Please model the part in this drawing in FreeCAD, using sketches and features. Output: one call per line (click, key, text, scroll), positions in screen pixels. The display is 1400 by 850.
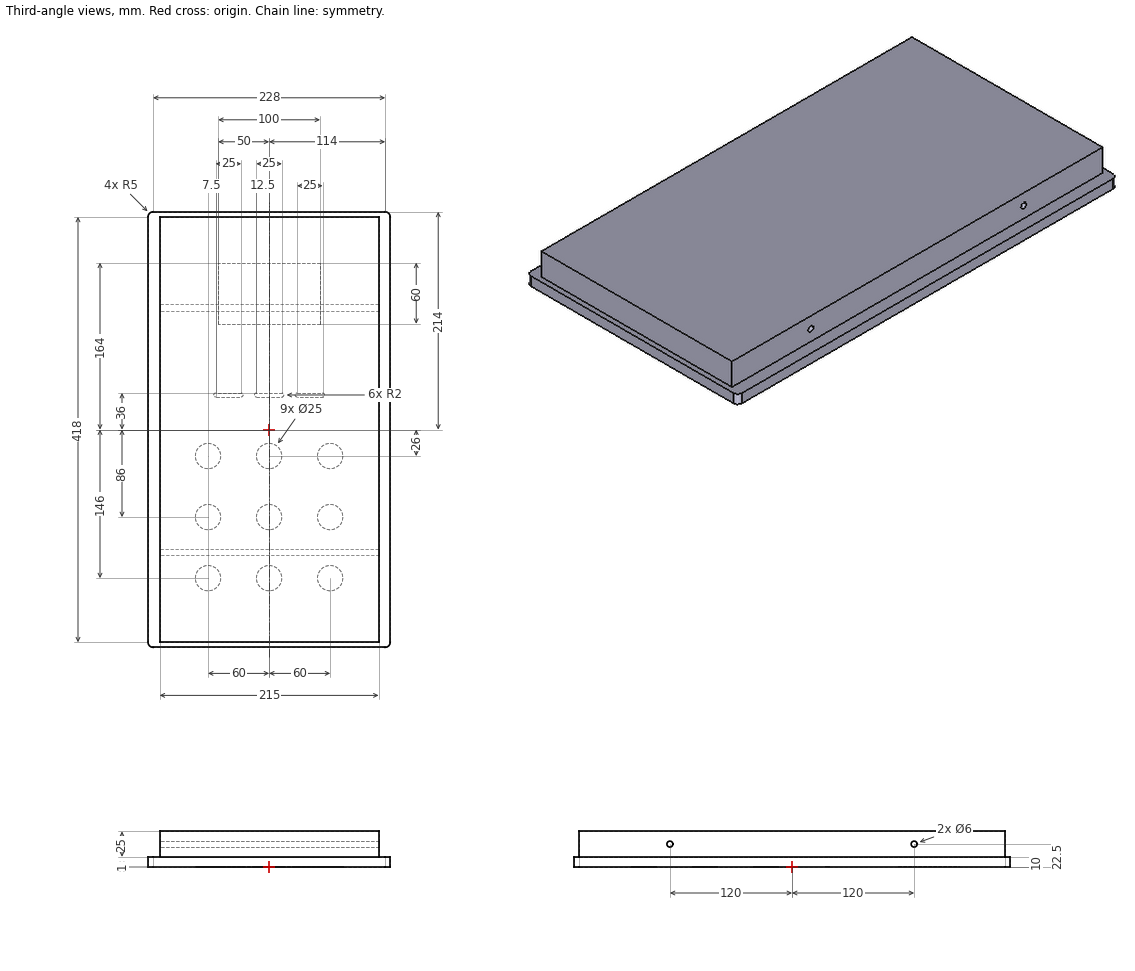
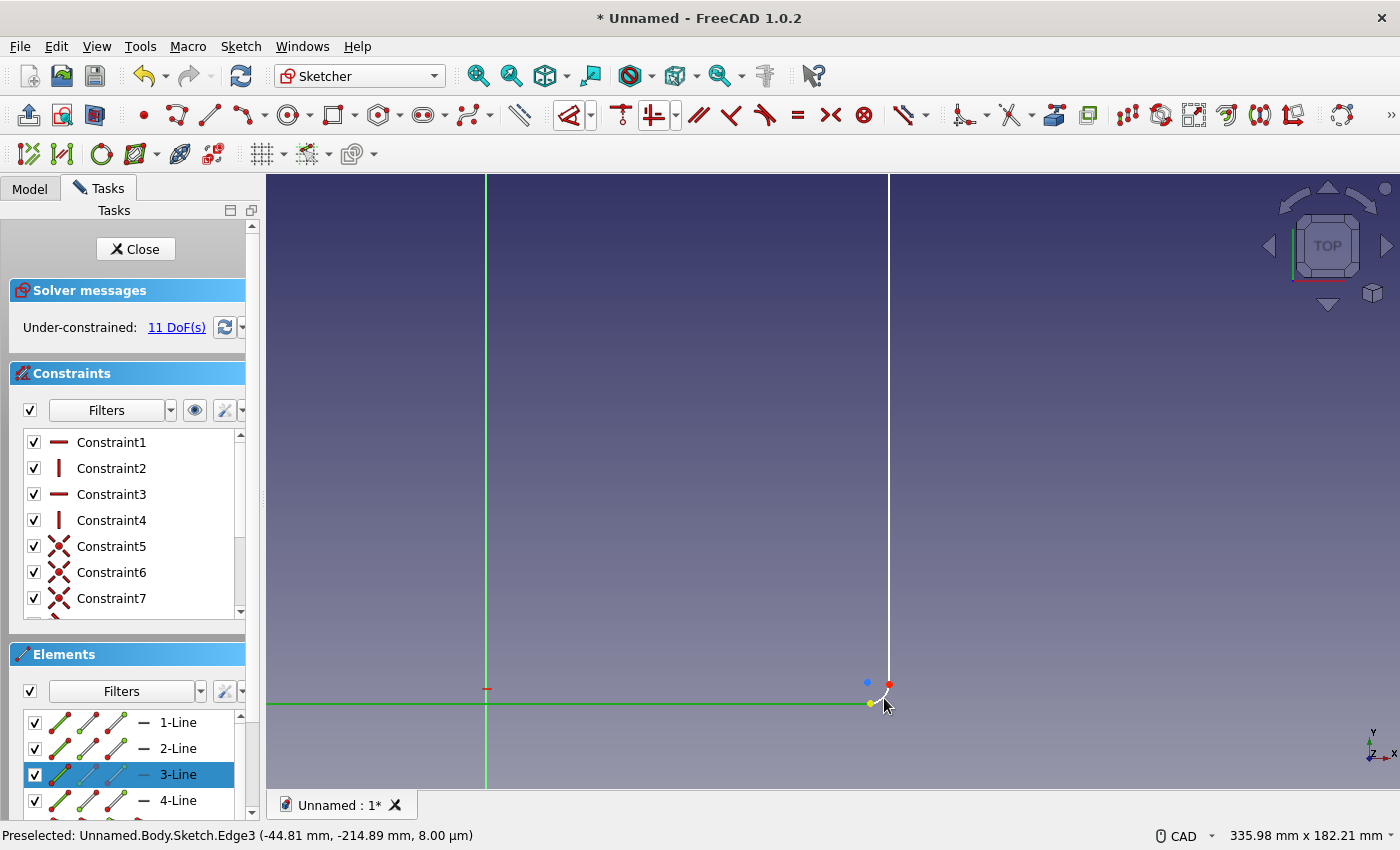
click(883, 698)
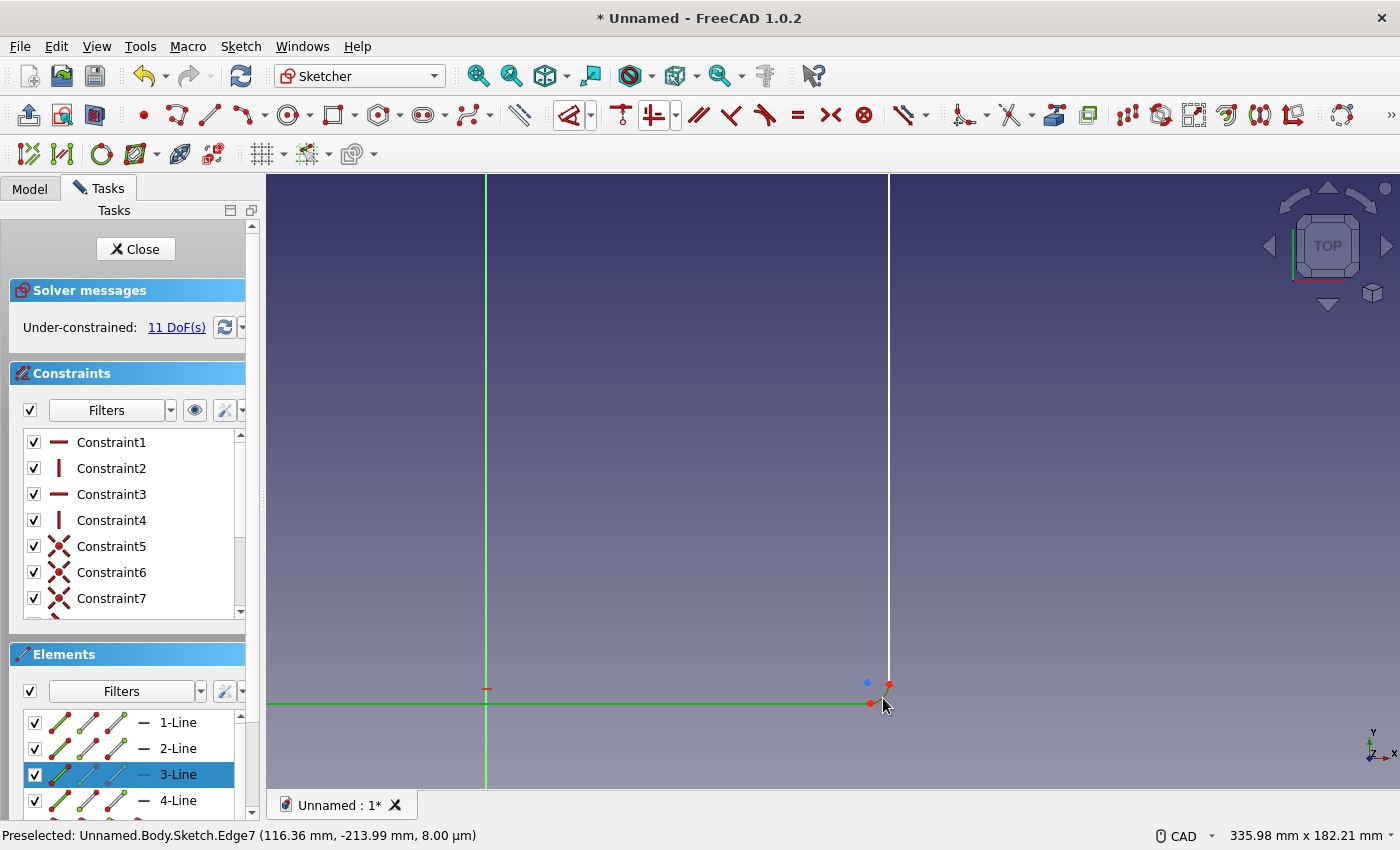
click(765, 116)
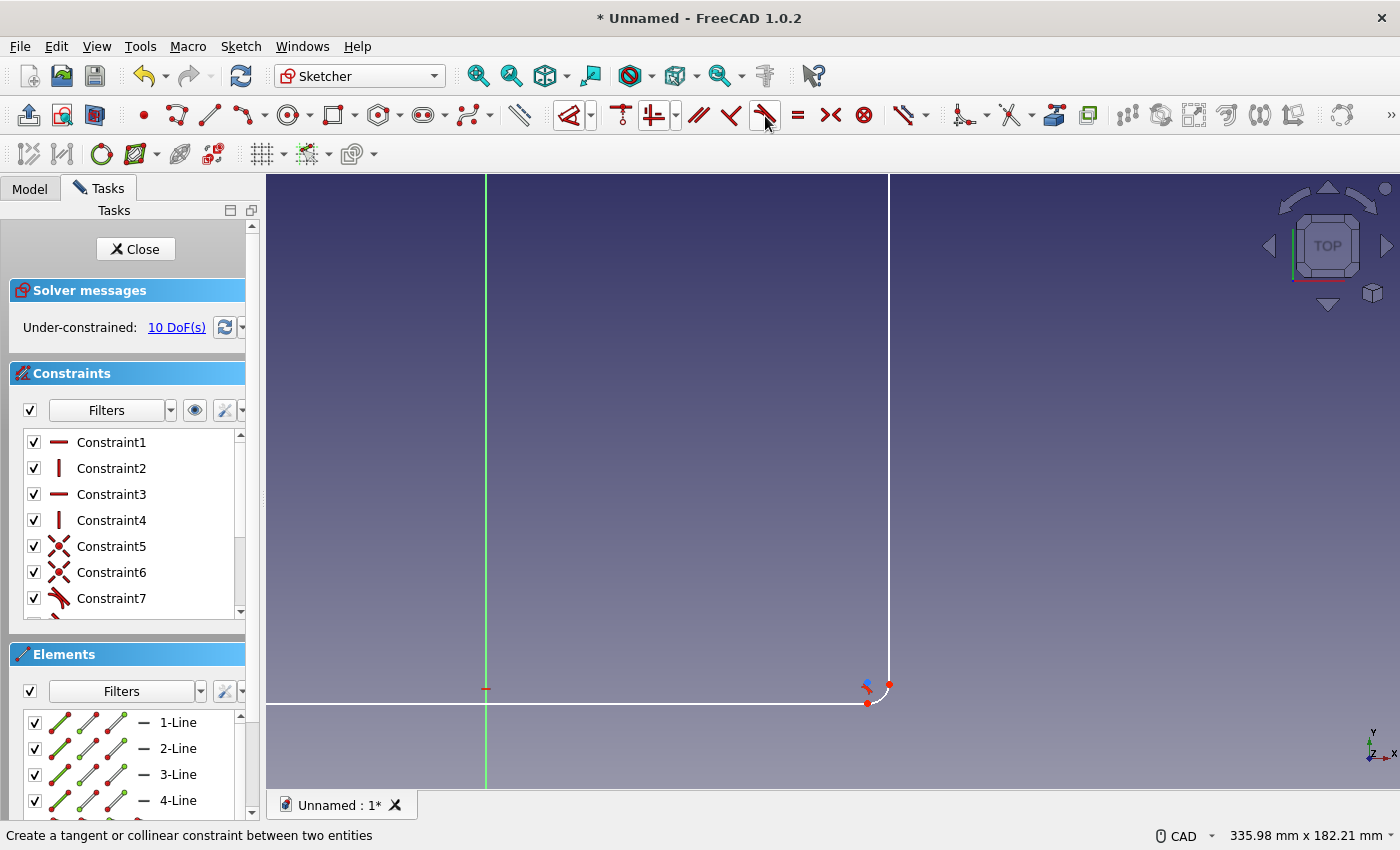
click(889, 262)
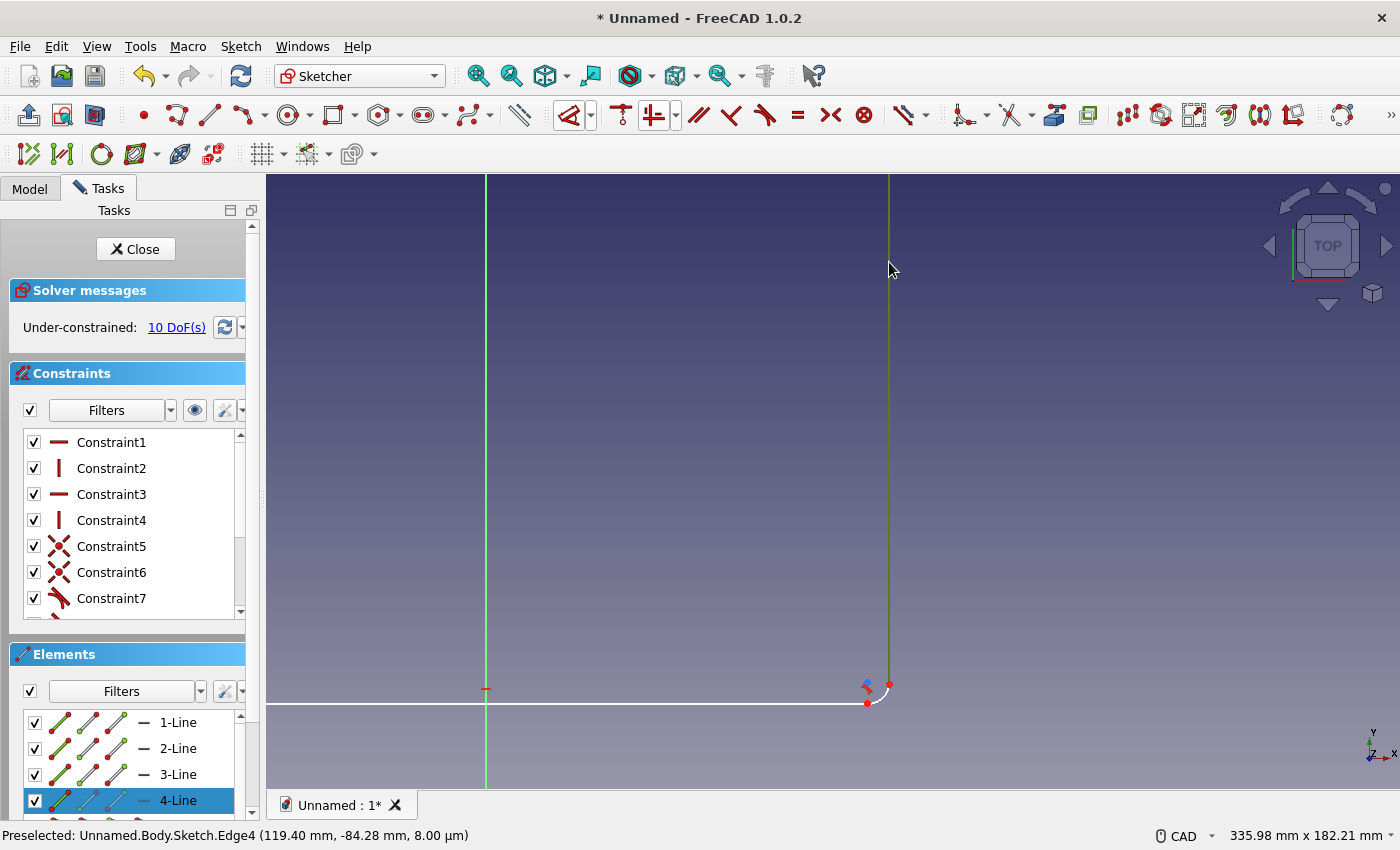
scroll(877, 702, up, 2)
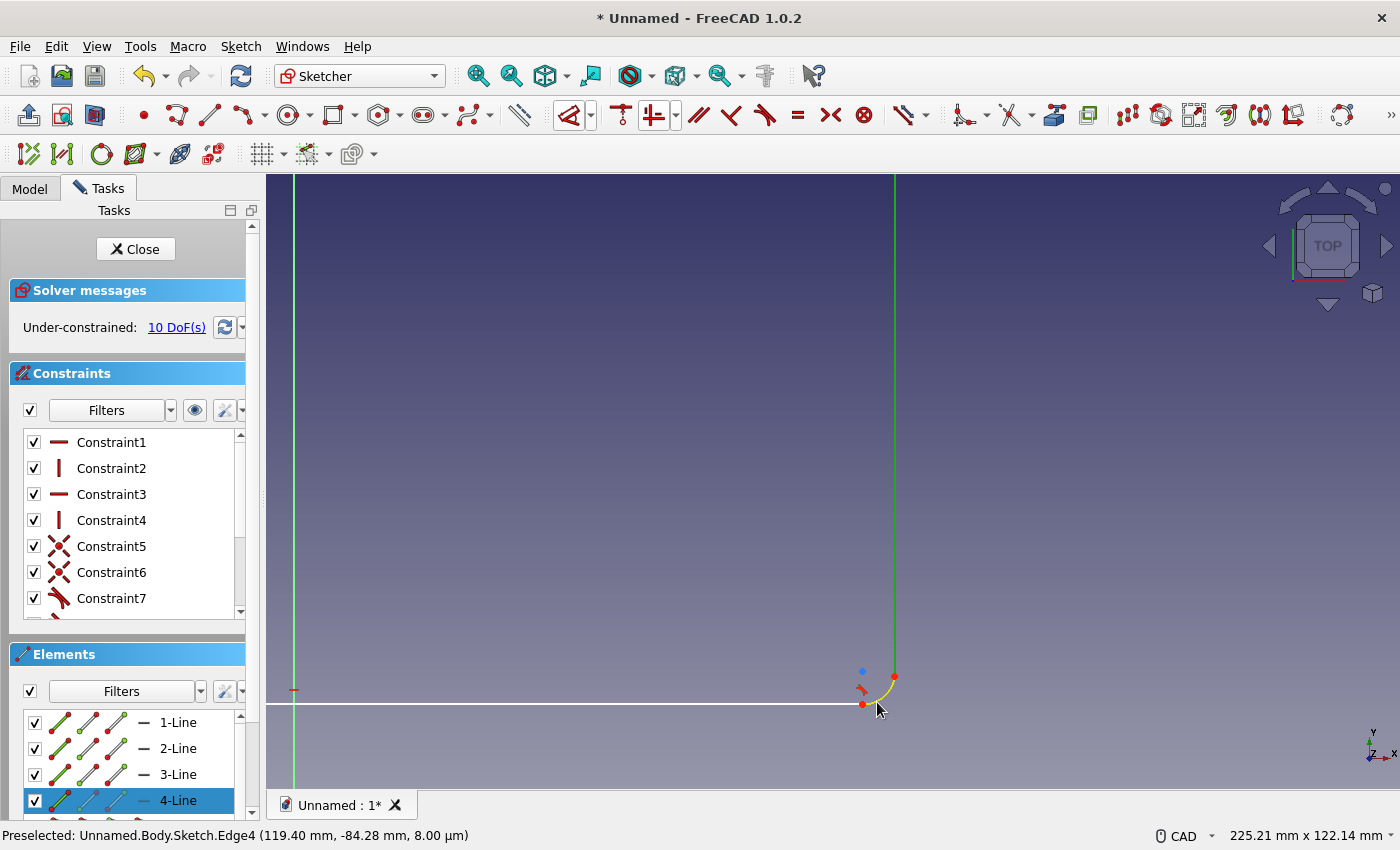
click(876, 701)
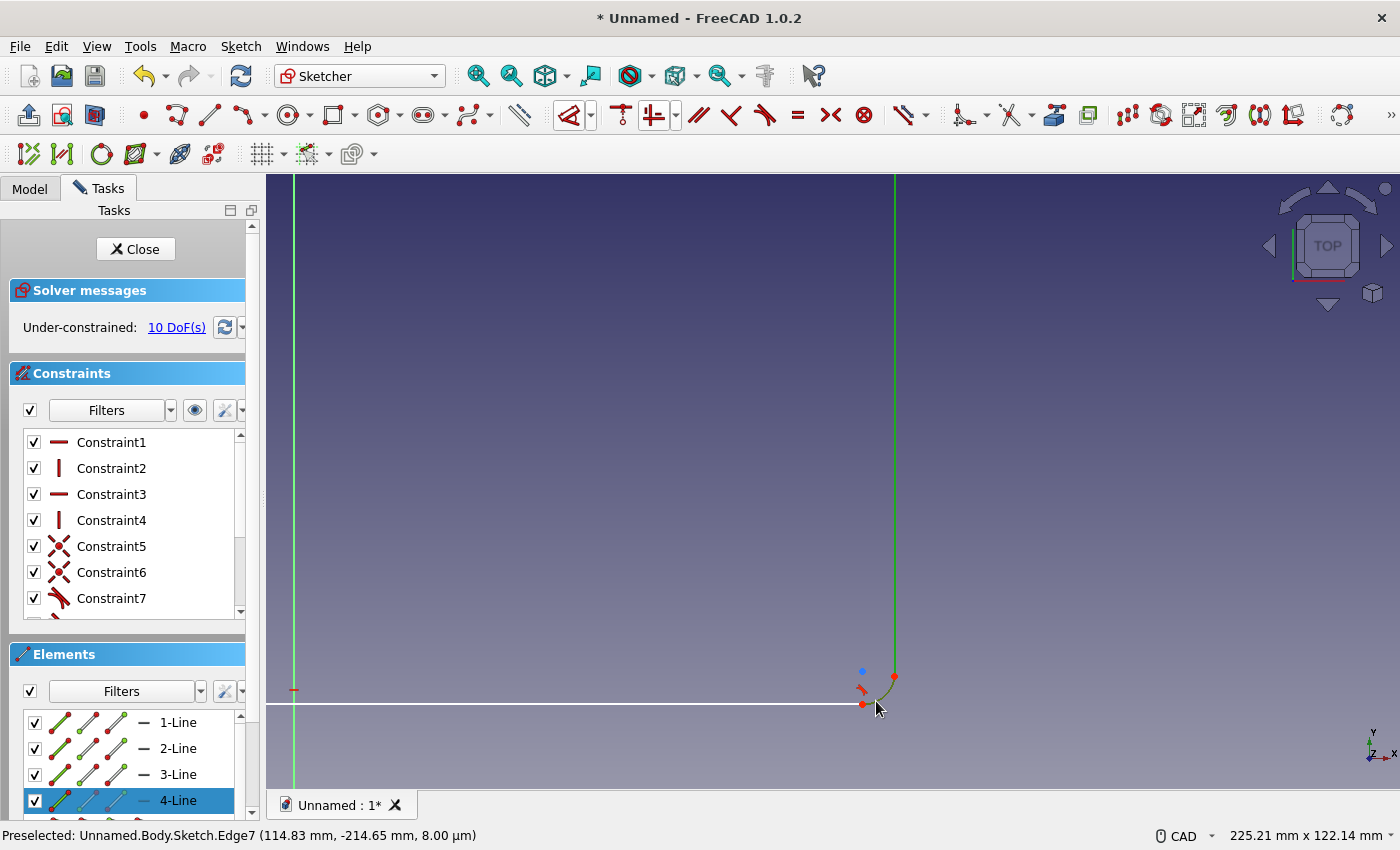
click(765, 116)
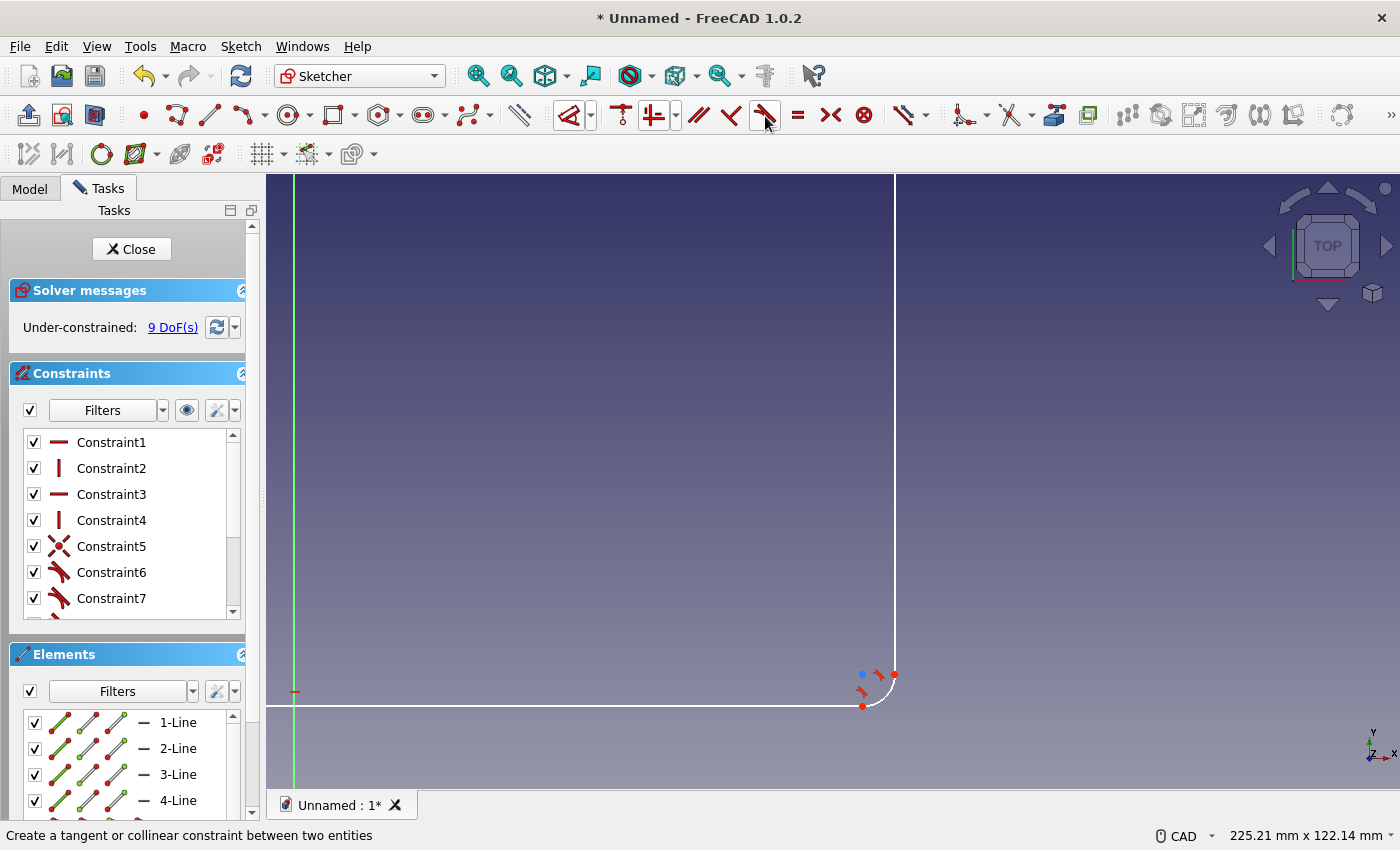
scroll(884, 699, down, 8)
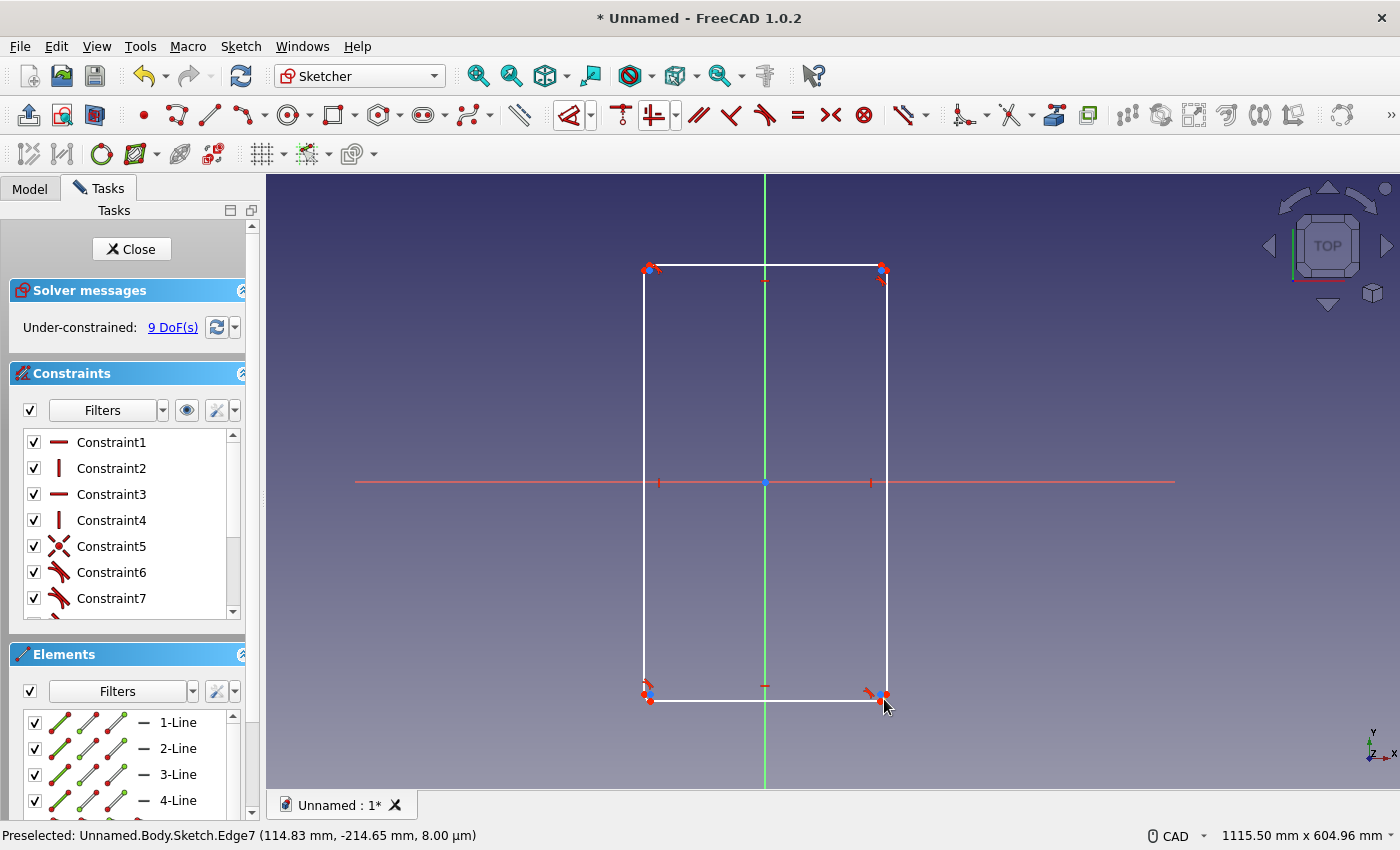
click(887, 610)